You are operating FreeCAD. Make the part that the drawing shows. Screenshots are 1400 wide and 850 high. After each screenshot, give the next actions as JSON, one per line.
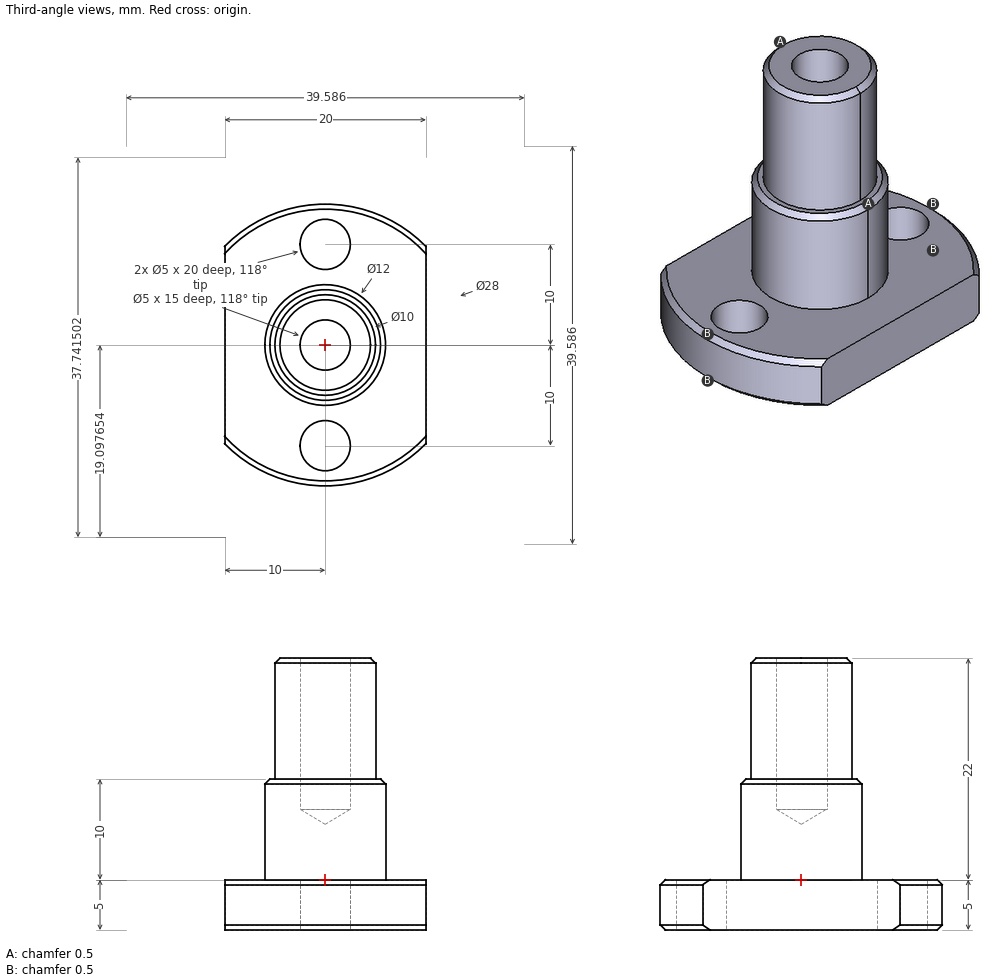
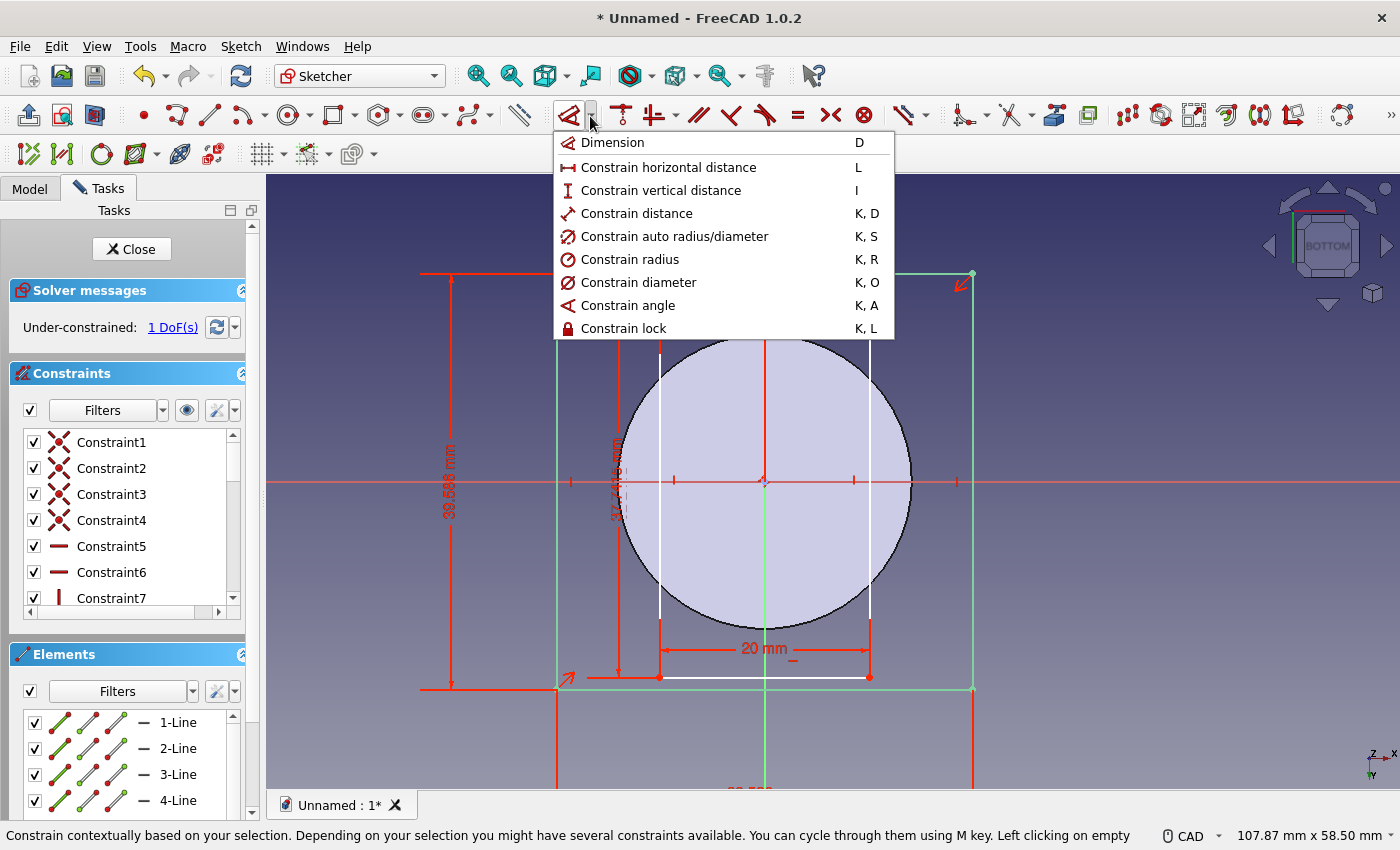
{"action": "left_click", "coordinate": [724, 190]}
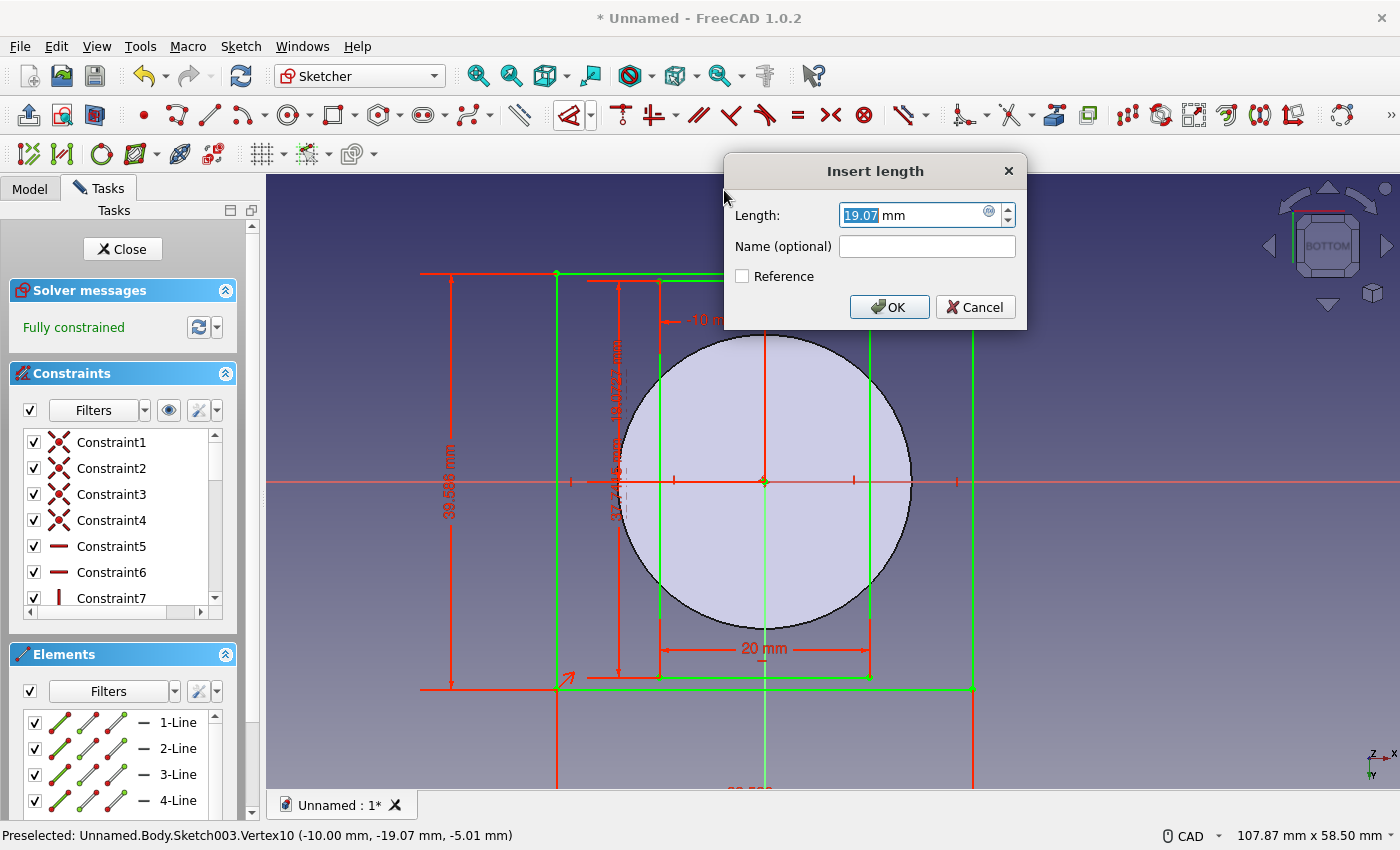
{"action": "type", "text": "19.097654"}
{"action": "key", "text": "Return"}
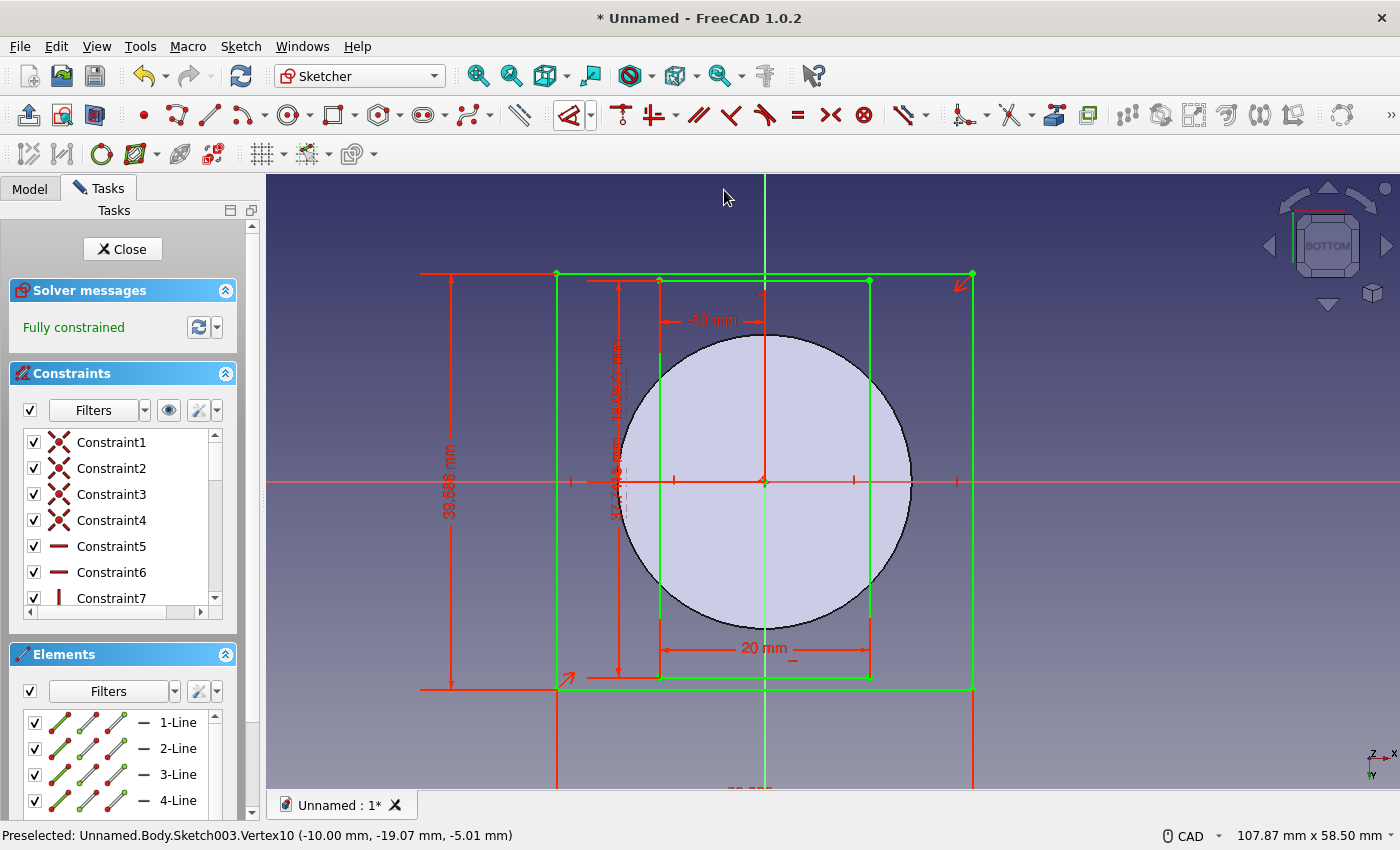
{"action": "left_click", "coordinate": [123, 249]}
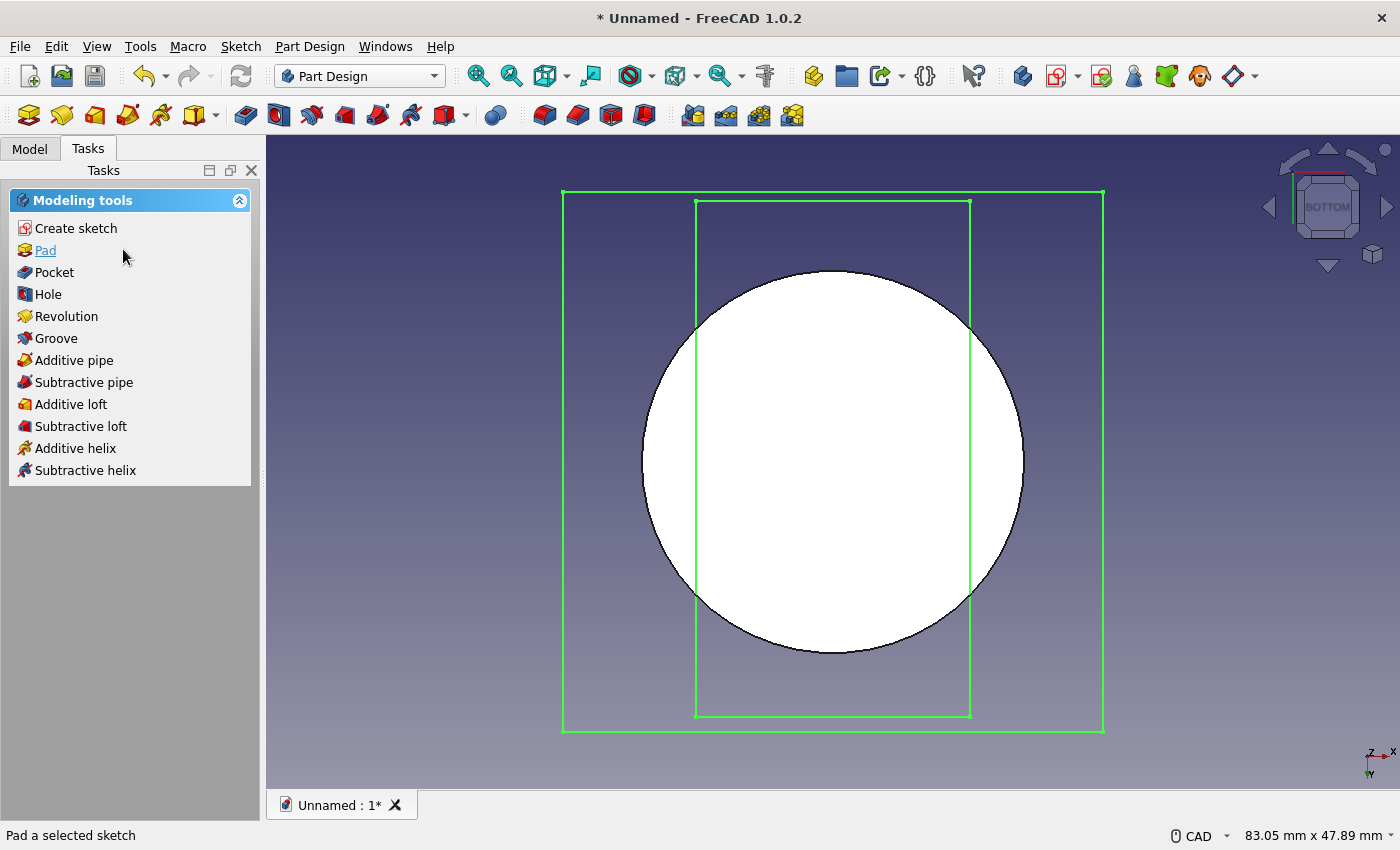
{"action": "left_click", "coordinate": [246, 116]}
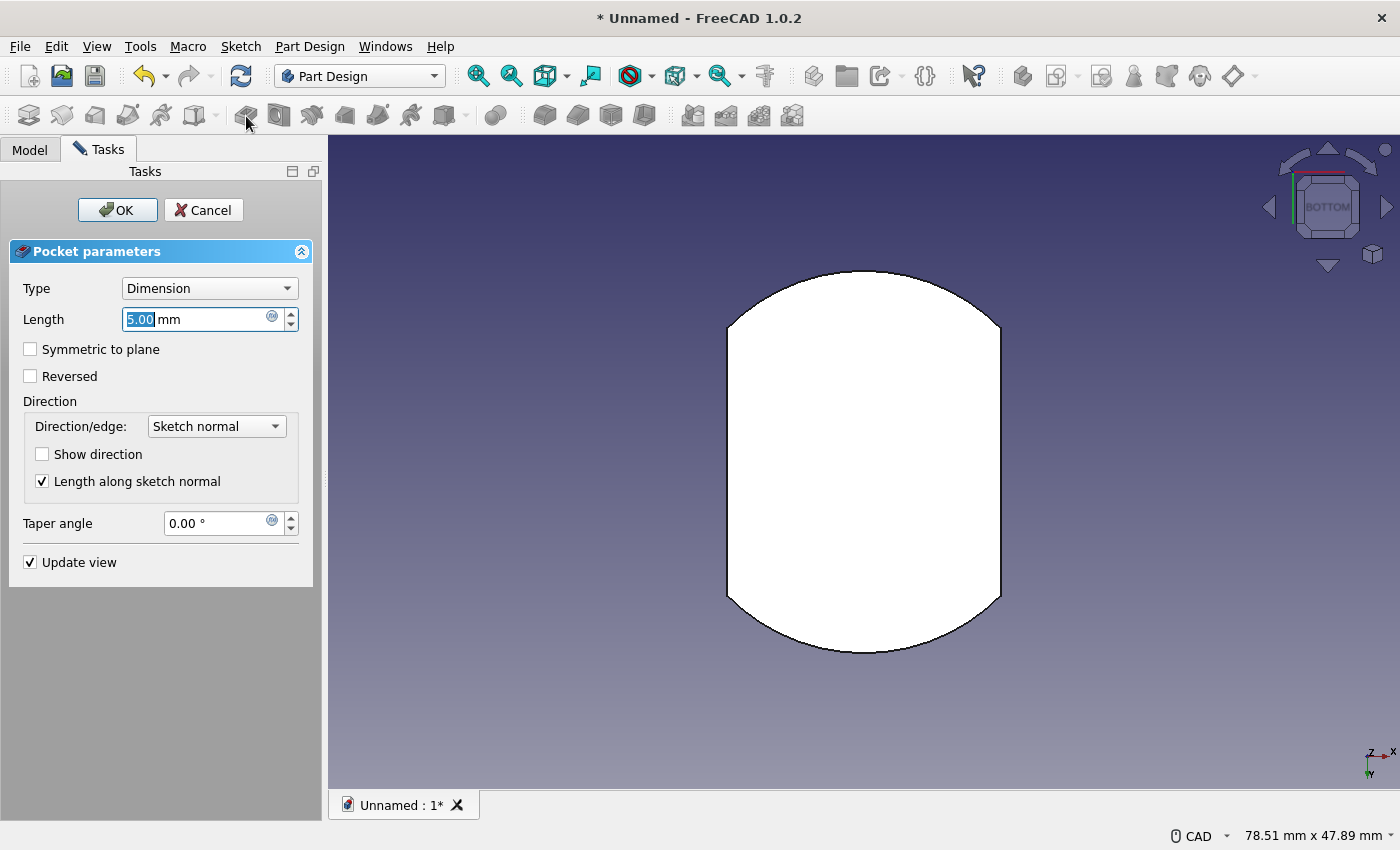
{"action": "type", "text": "5"}
{"action": "key", "text": "Tab"}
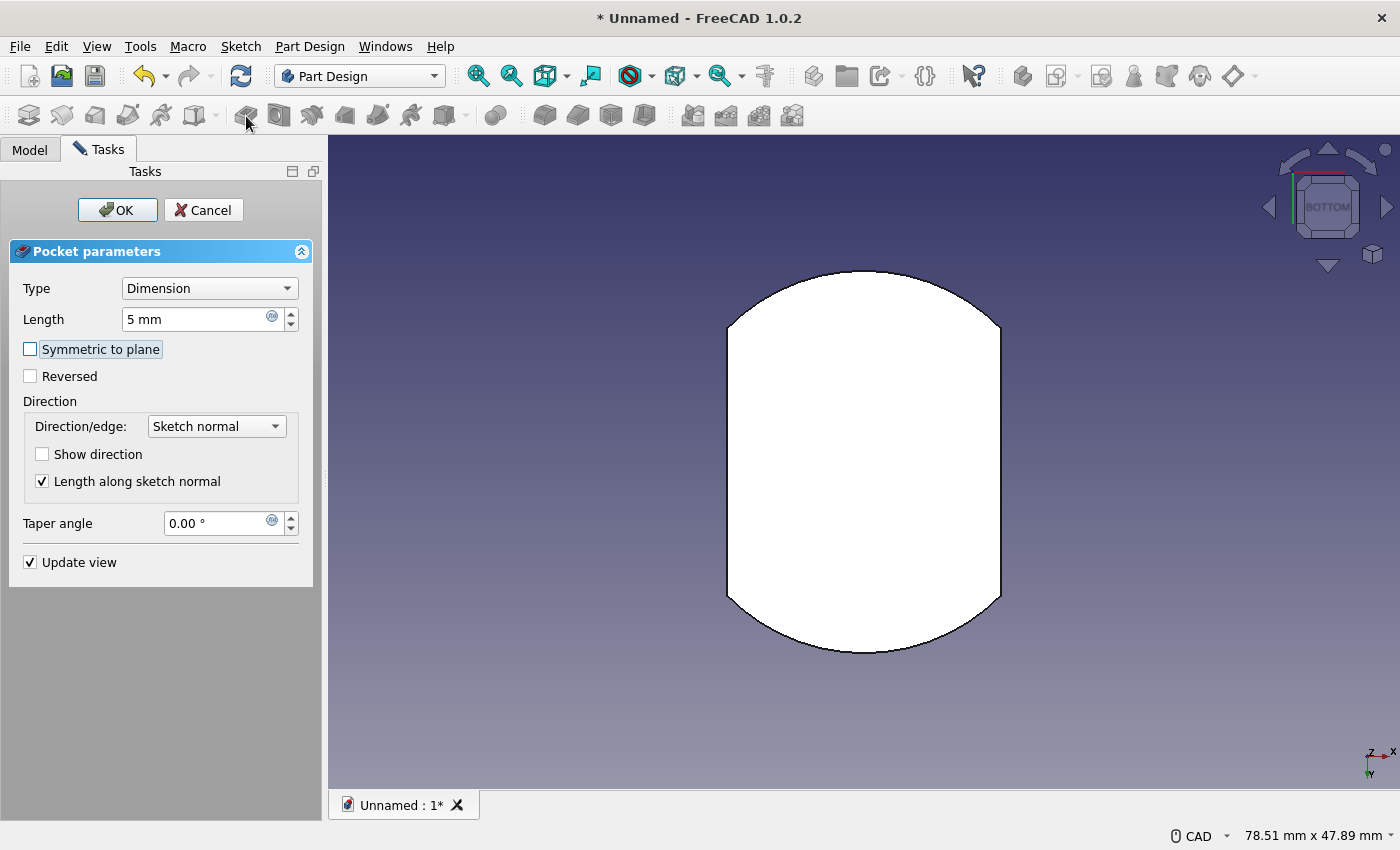
{"action": "left_click", "coordinate": [118, 210]}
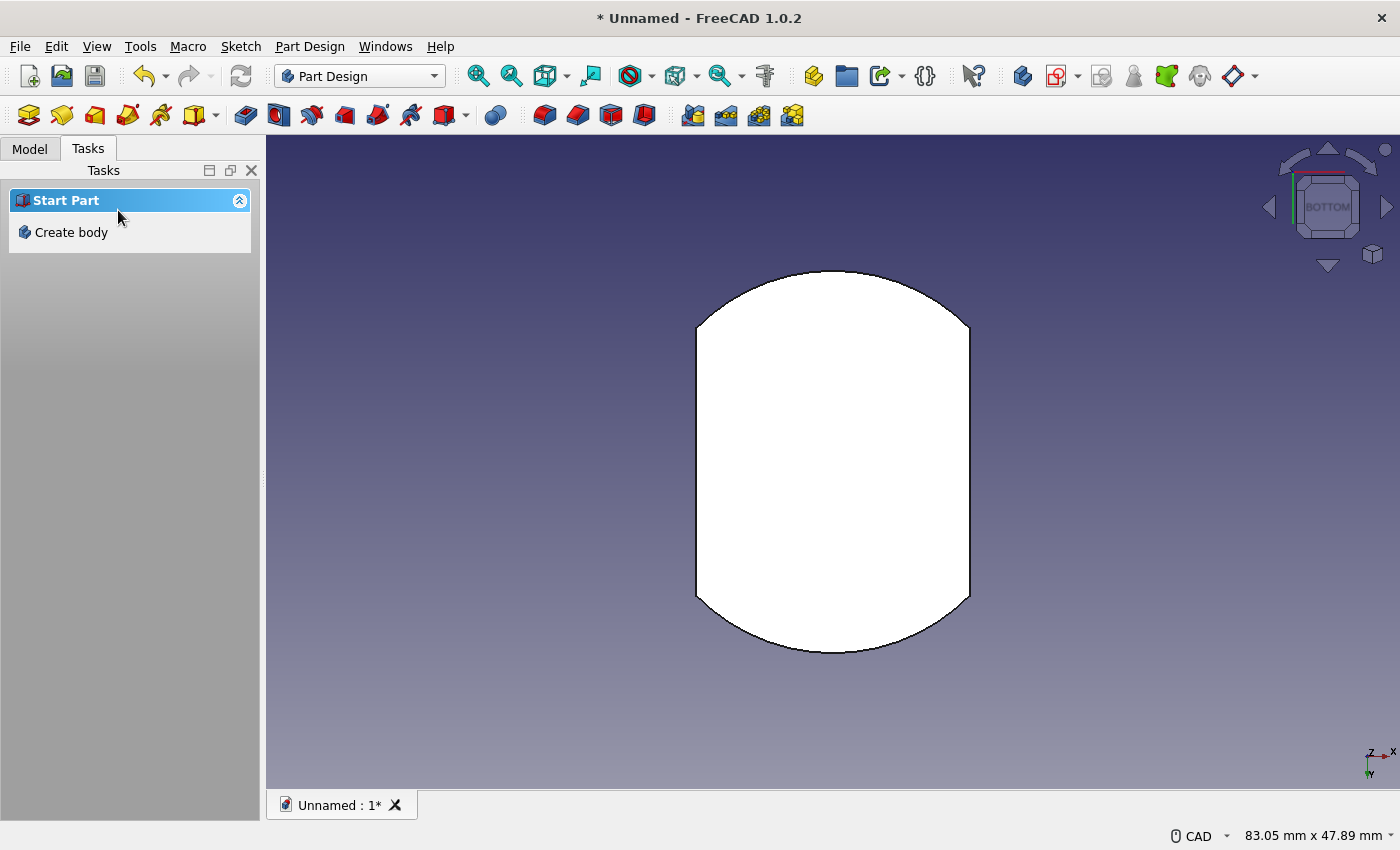
{"action": "left_click", "coordinate": [1056, 76]}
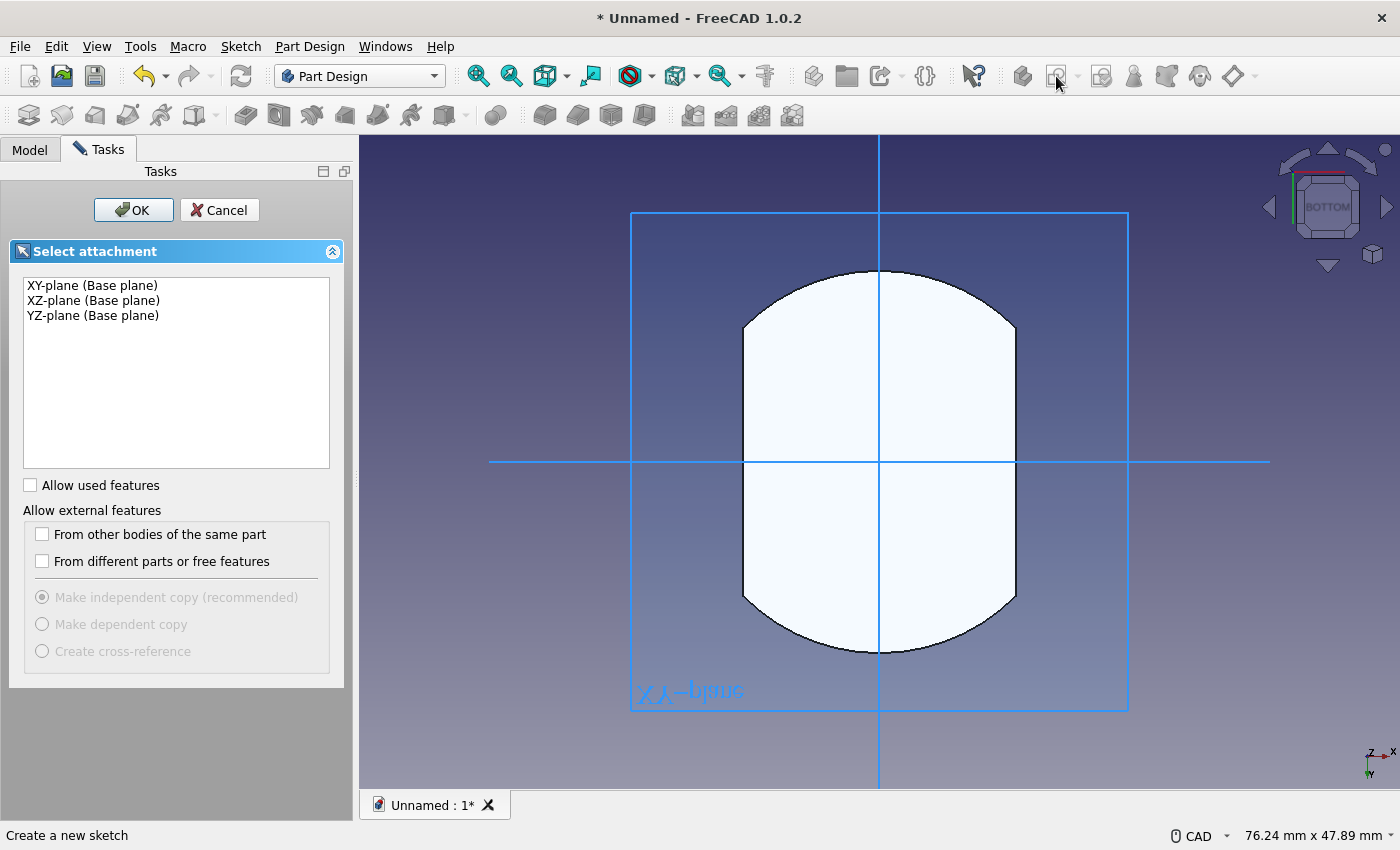
{"action": "left_click", "coordinate": [84, 286]}